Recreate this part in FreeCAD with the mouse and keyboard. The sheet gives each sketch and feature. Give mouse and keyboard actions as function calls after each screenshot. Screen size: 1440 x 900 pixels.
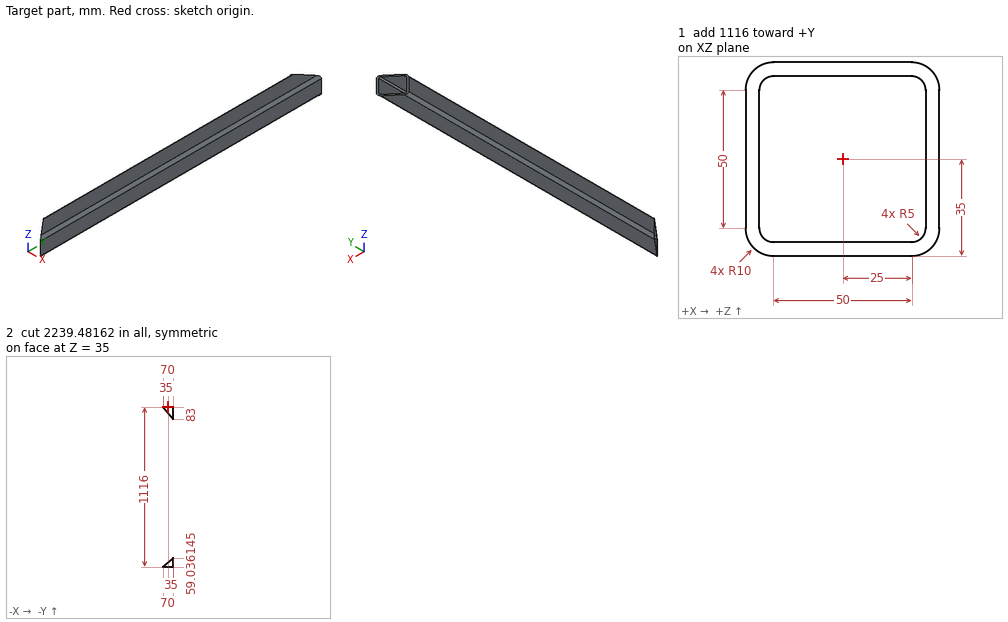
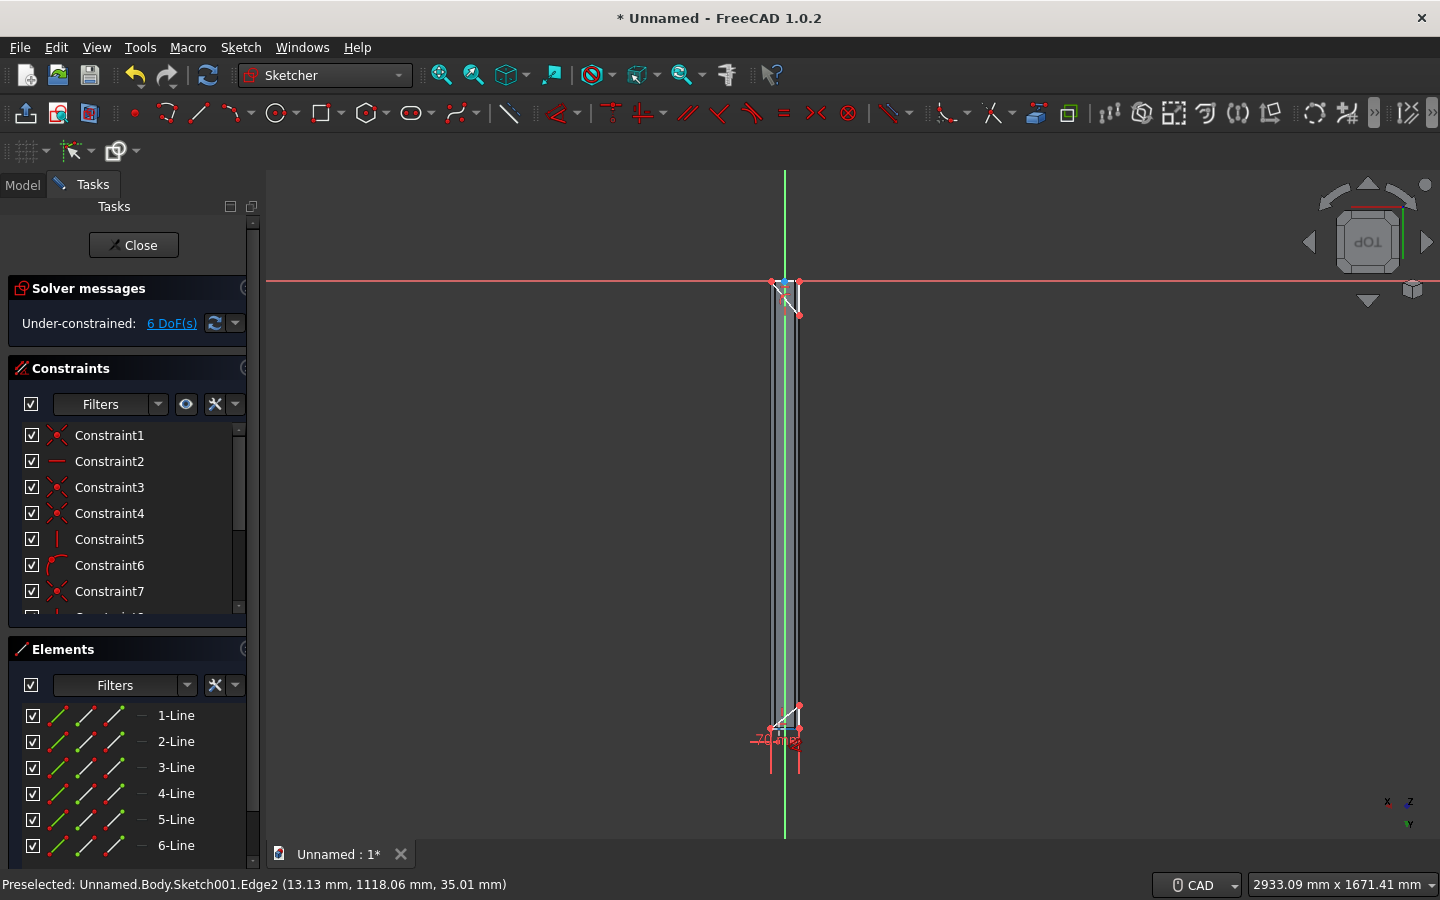
scroll(799, 306, up, 4)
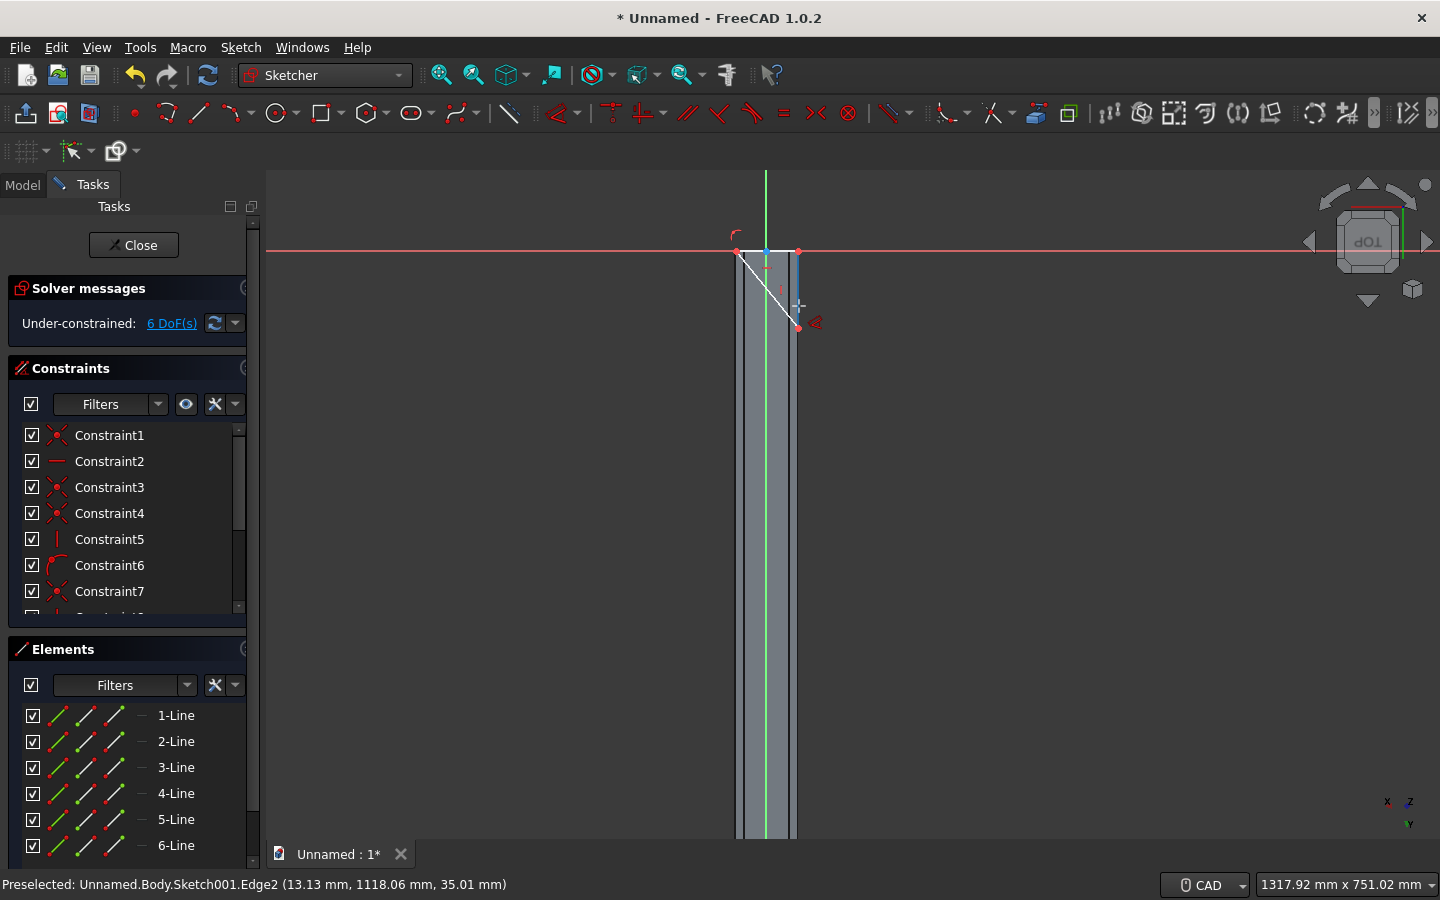
click(798, 305)
click(832, 290)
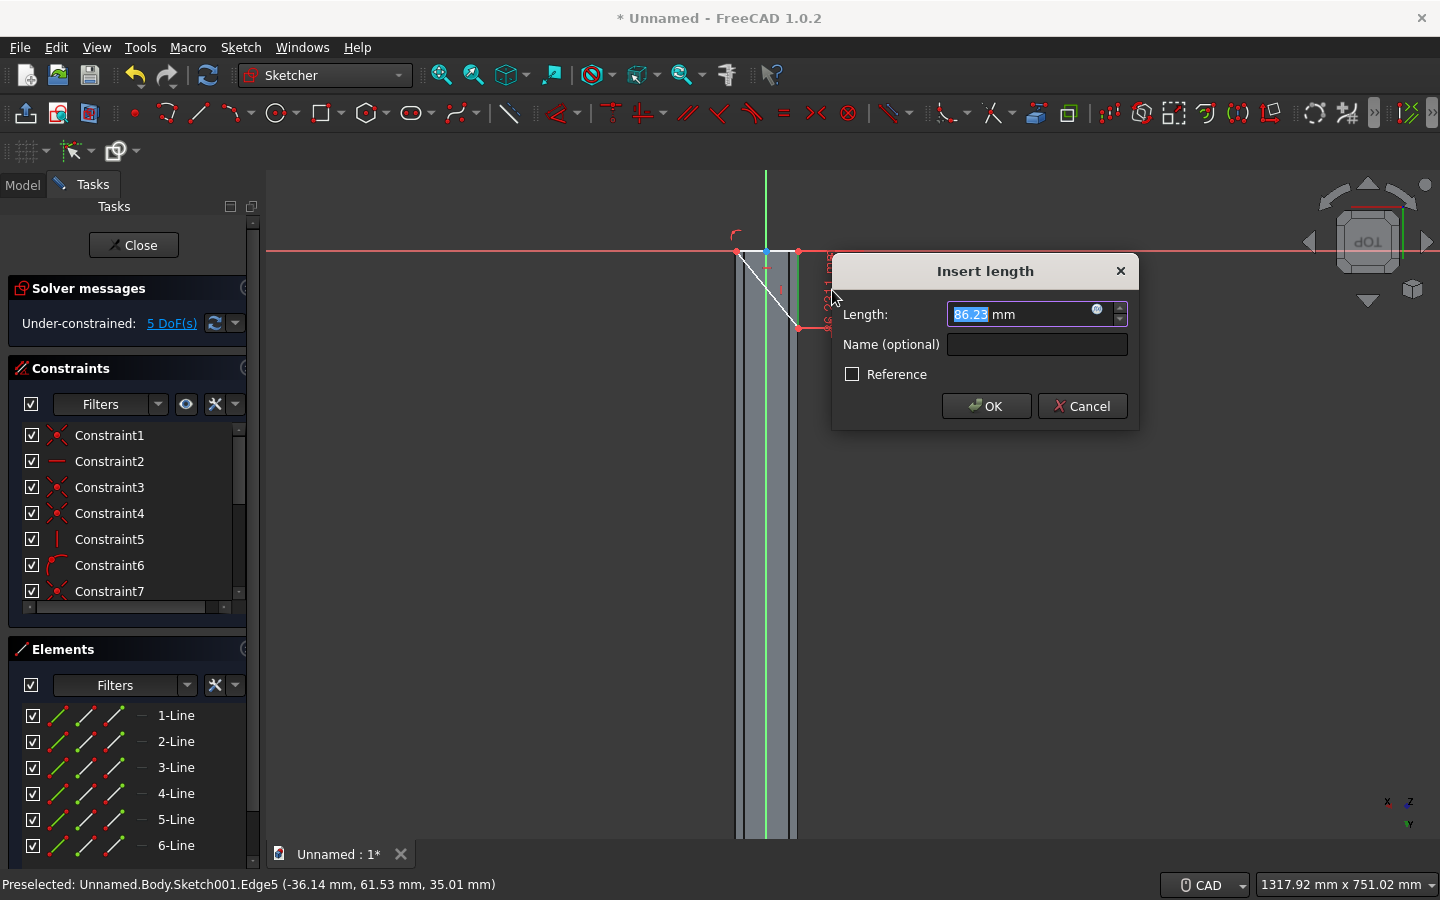
text(83)
key(Return)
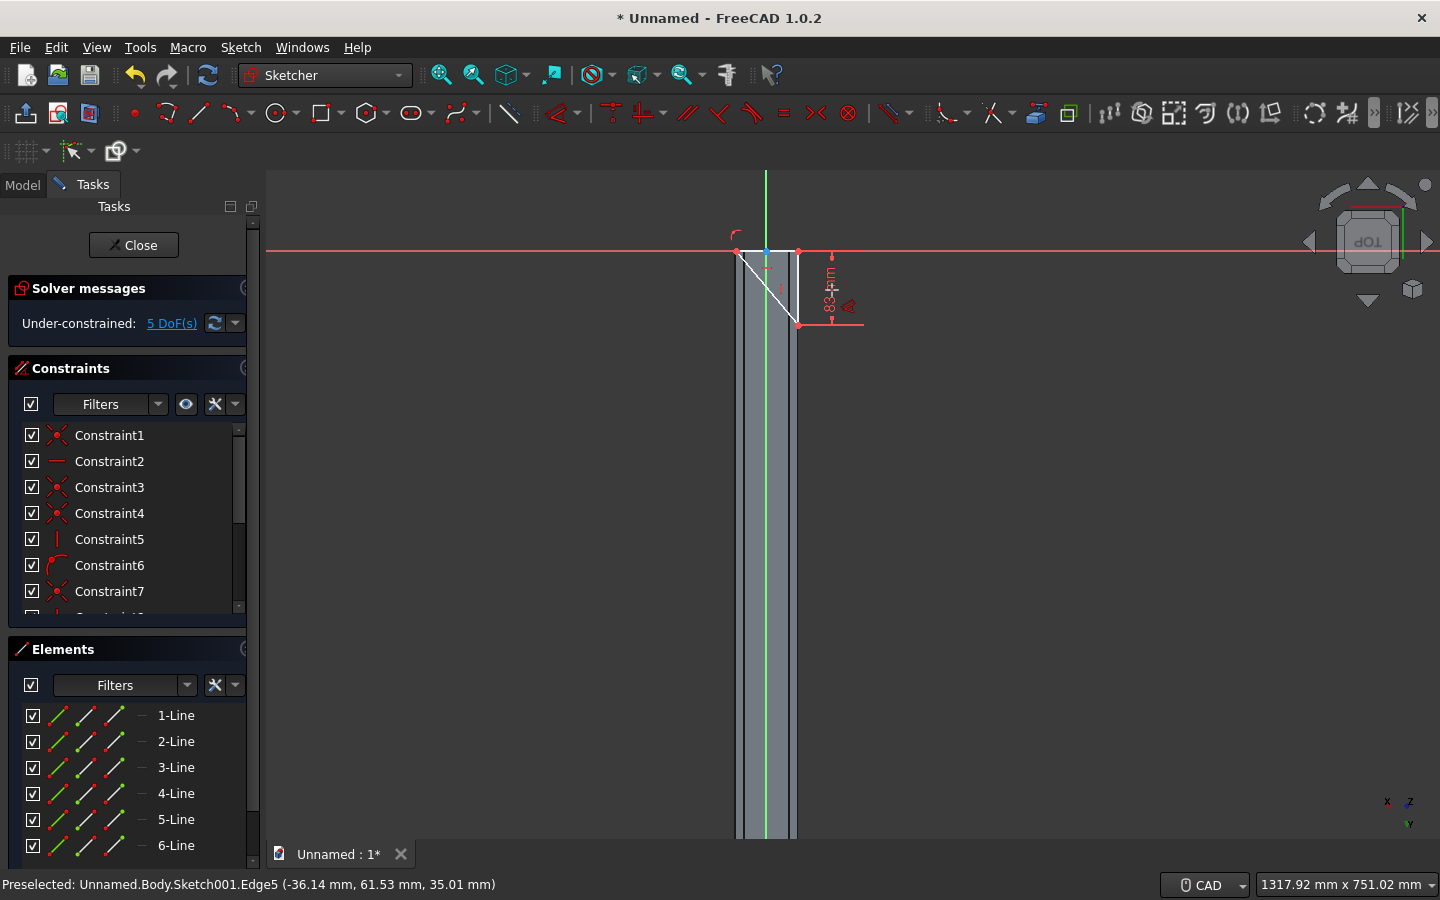
click(780, 251)
click(753, 217)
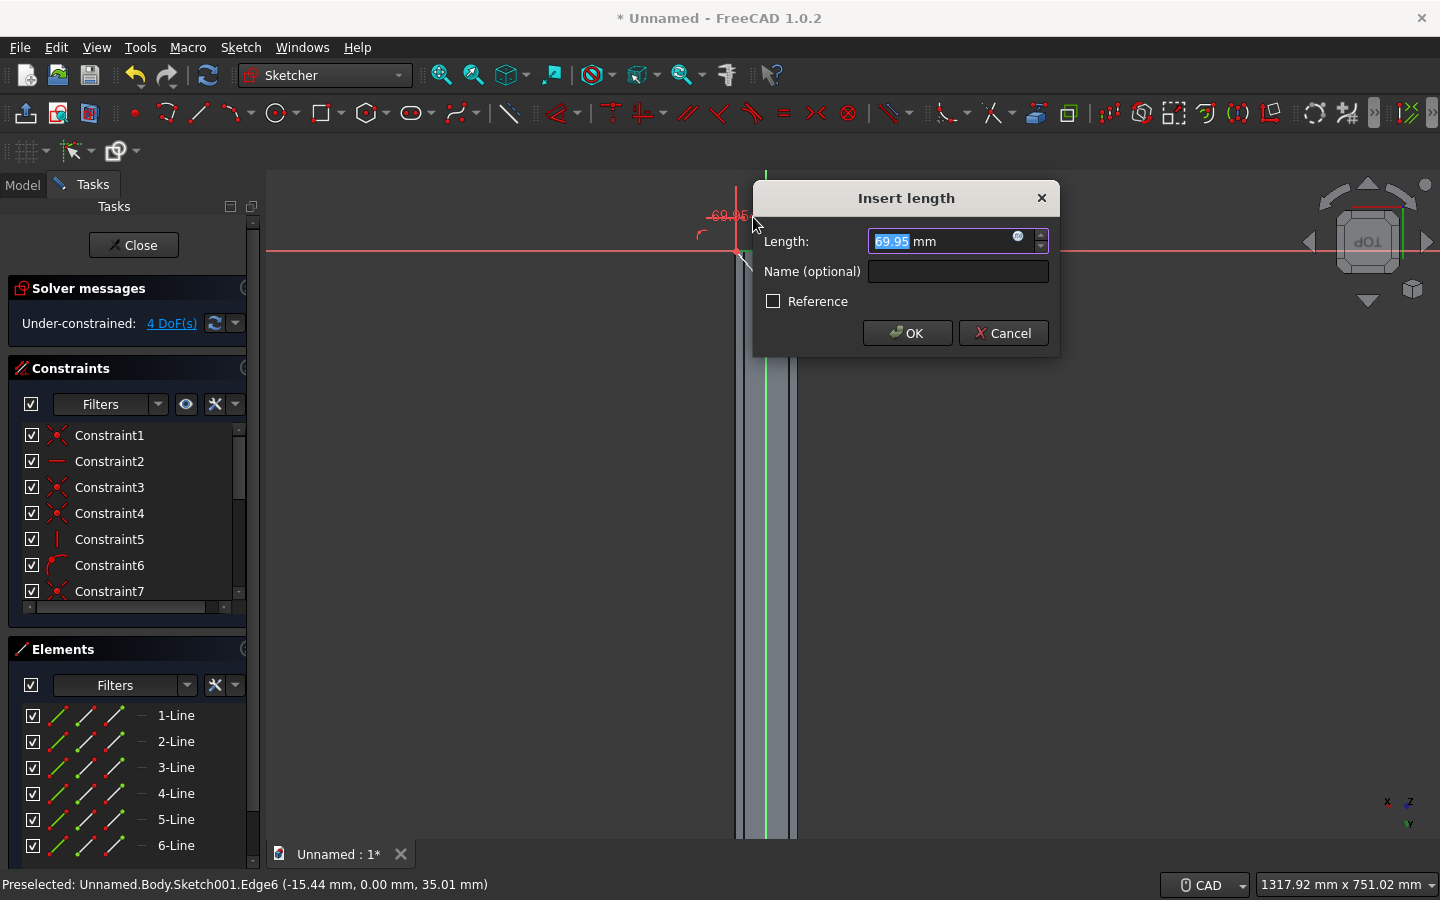
text(70)
key(Return)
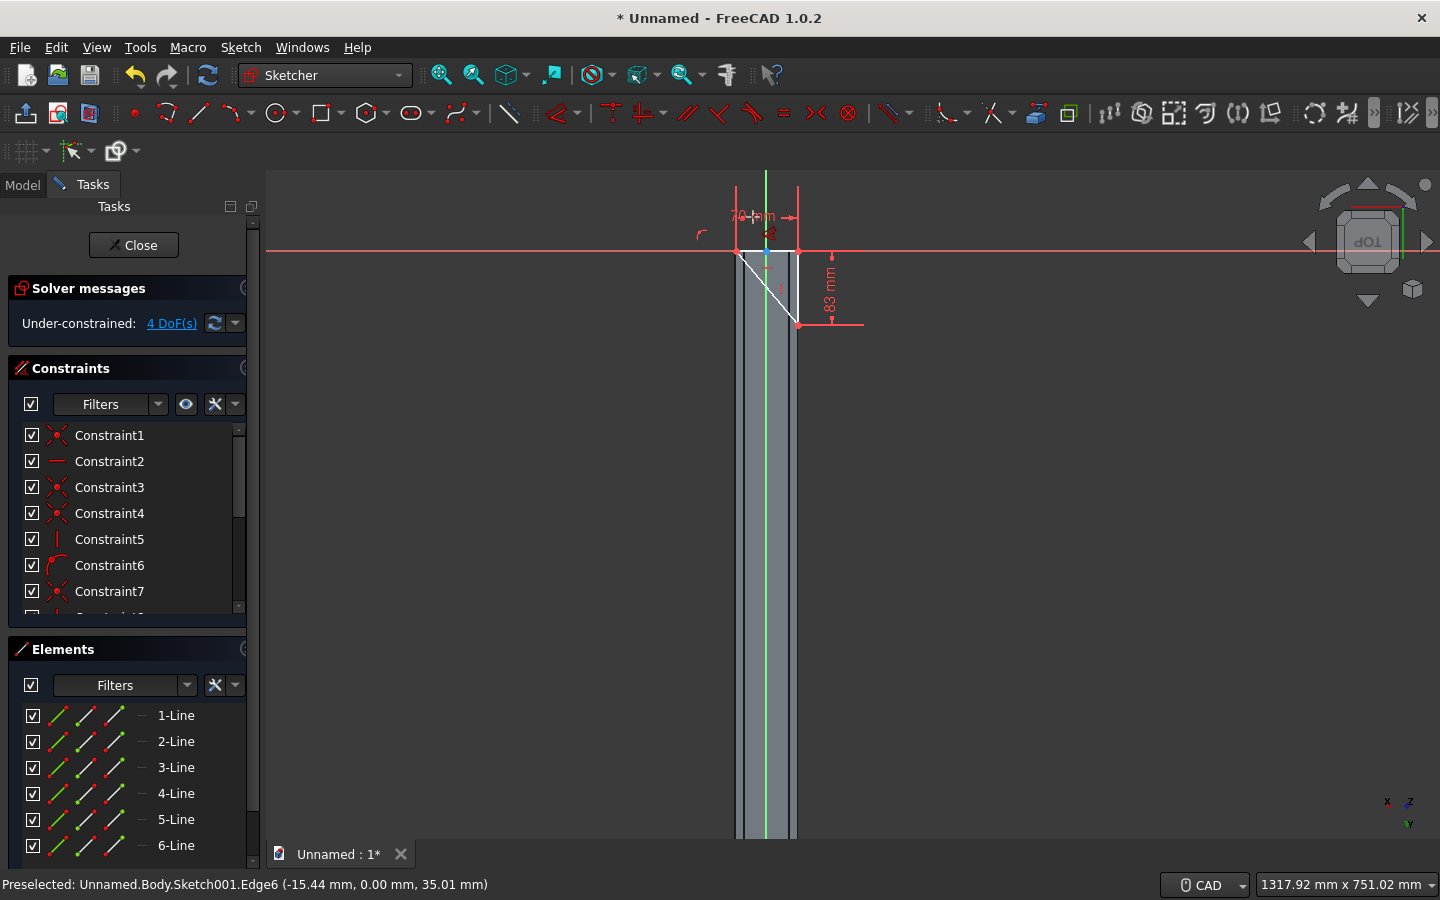
scroll(799, 306, down, 4)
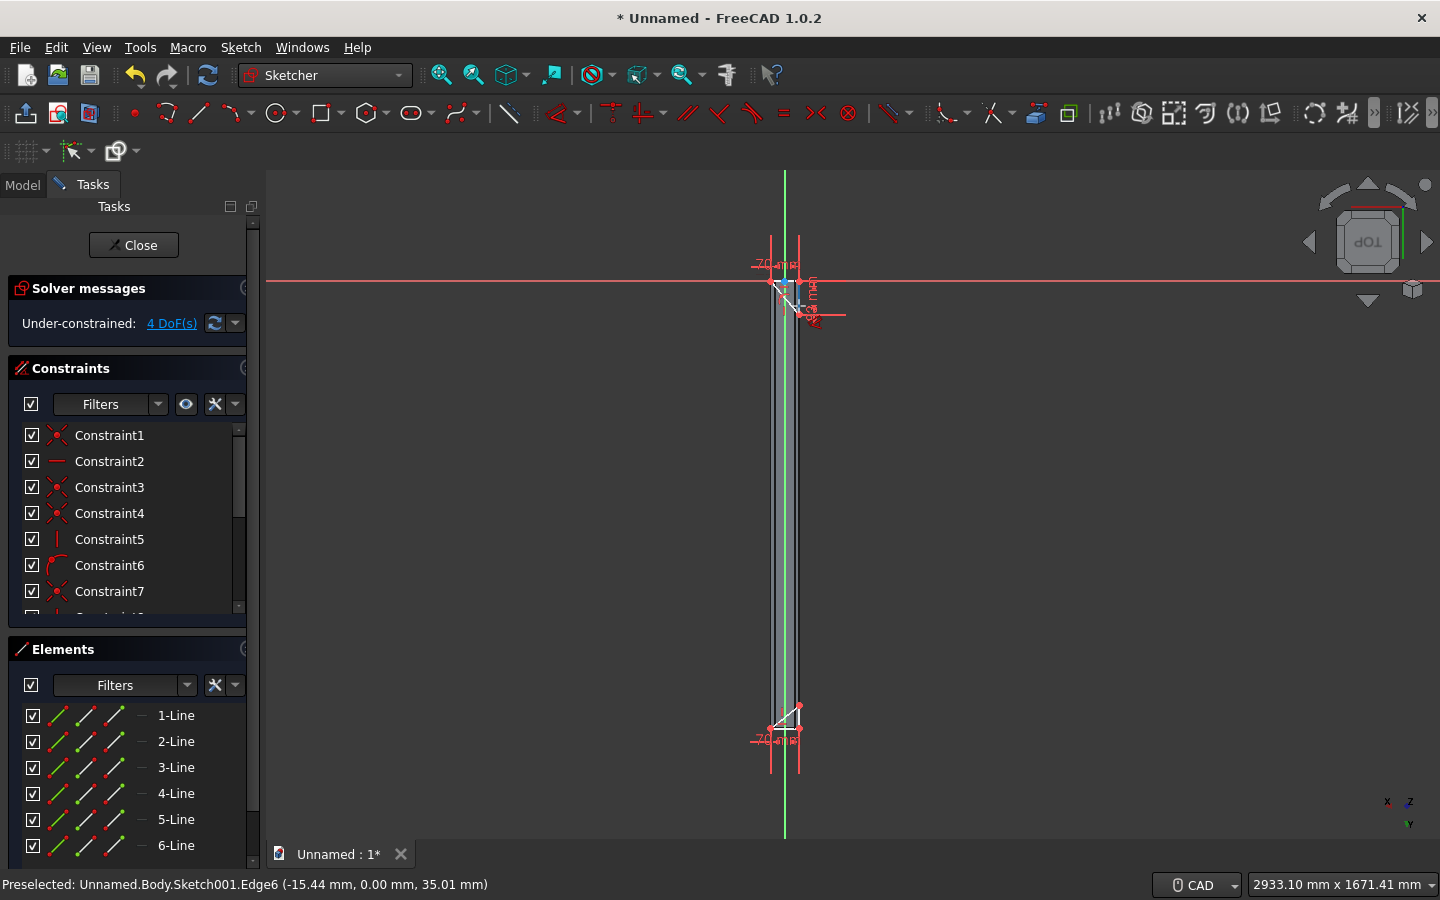
scroll(799, 706, up, 6)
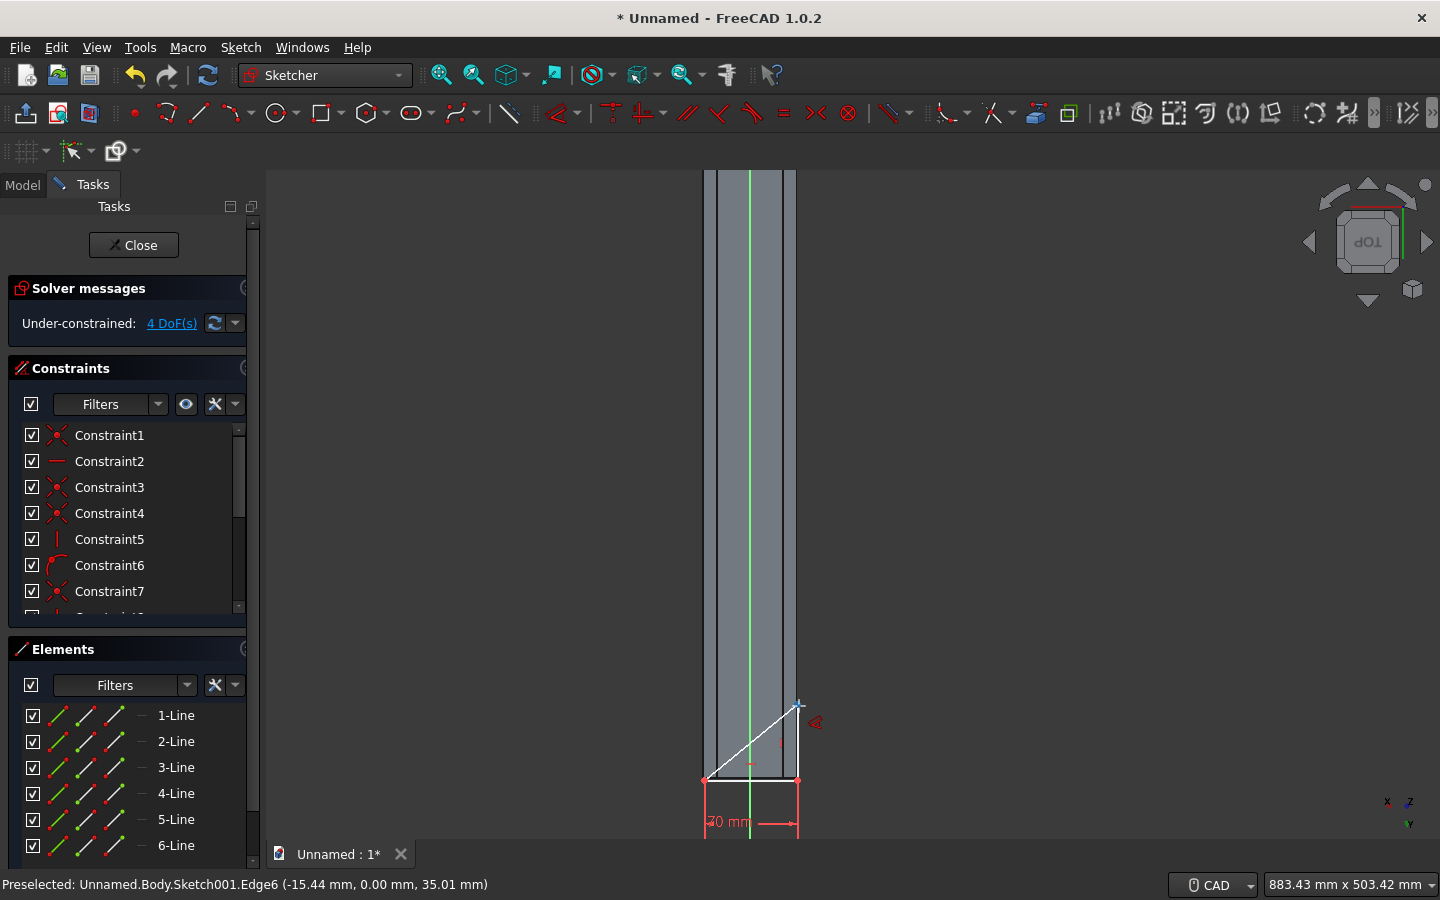
click(798, 704)
click(774, 762)